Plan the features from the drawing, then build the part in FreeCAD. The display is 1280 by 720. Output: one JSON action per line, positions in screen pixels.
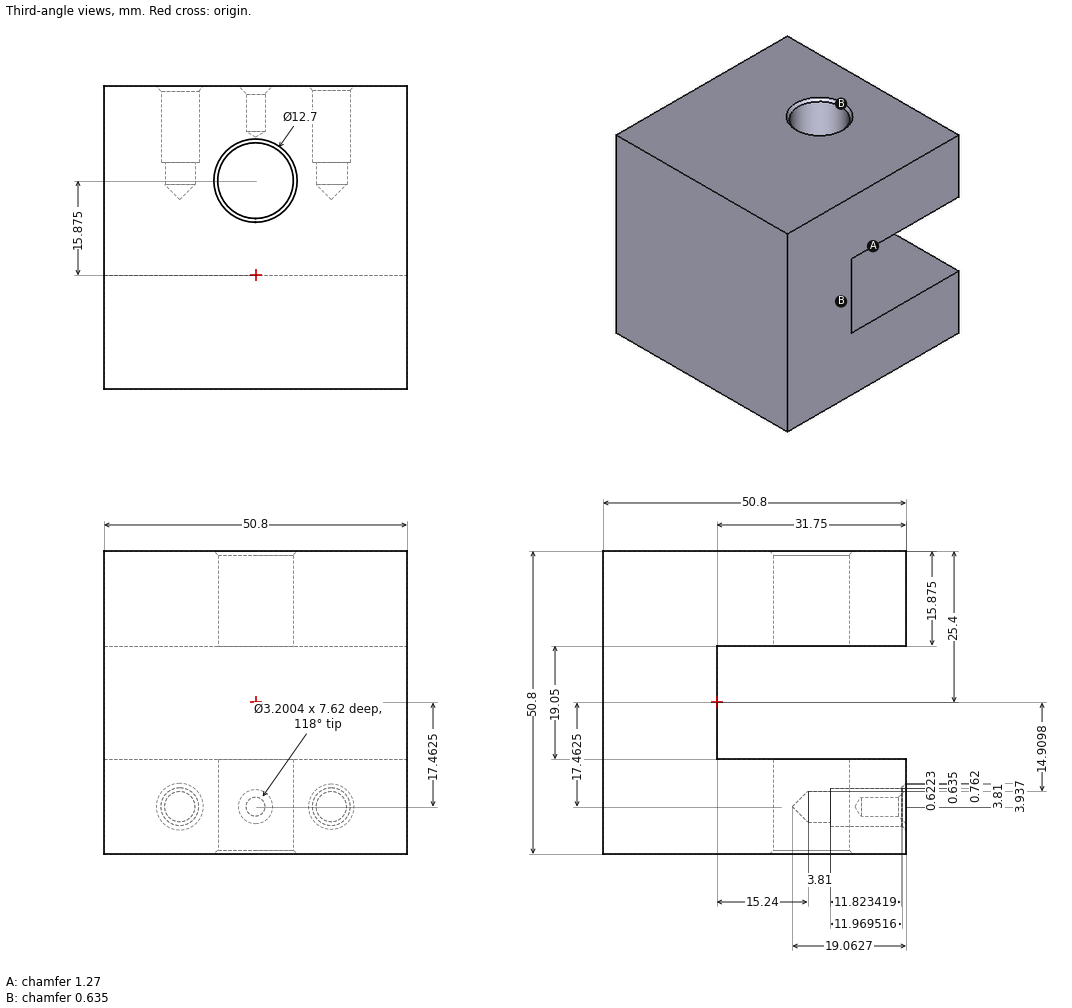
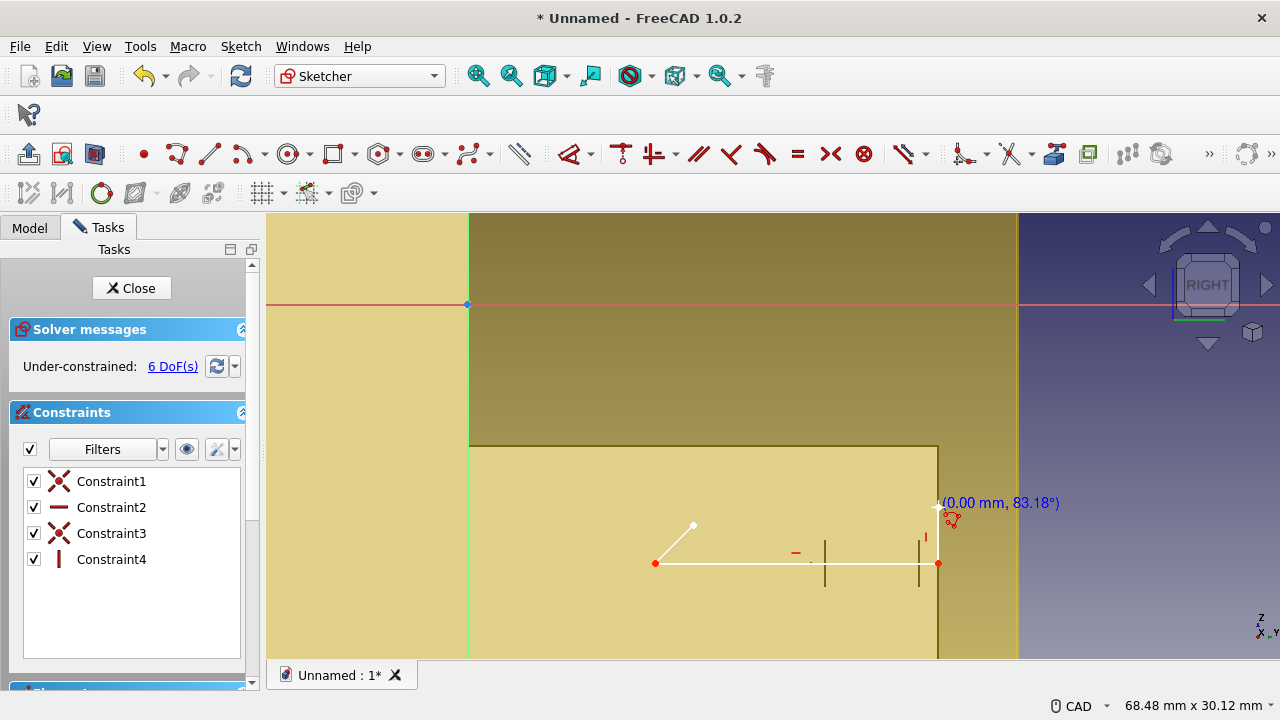
{"action": "scroll", "coordinate": [927, 516], "scroll_direction": "up", "scroll_amount": 2}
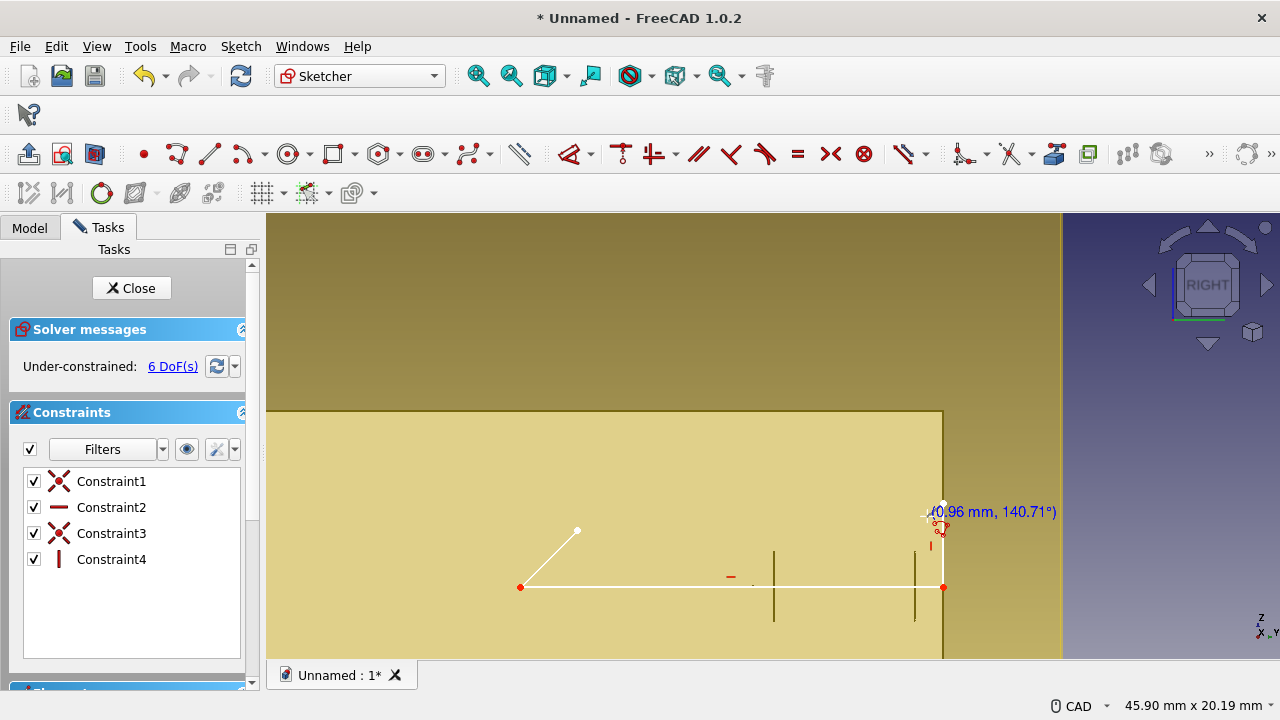
{"action": "left_click", "coordinate": [927, 516]}
{"action": "left_click", "coordinate": [662, 516]}
{"action": "left_click", "coordinate": [662, 530]}
{"action": "left_click", "coordinate": [578, 531]}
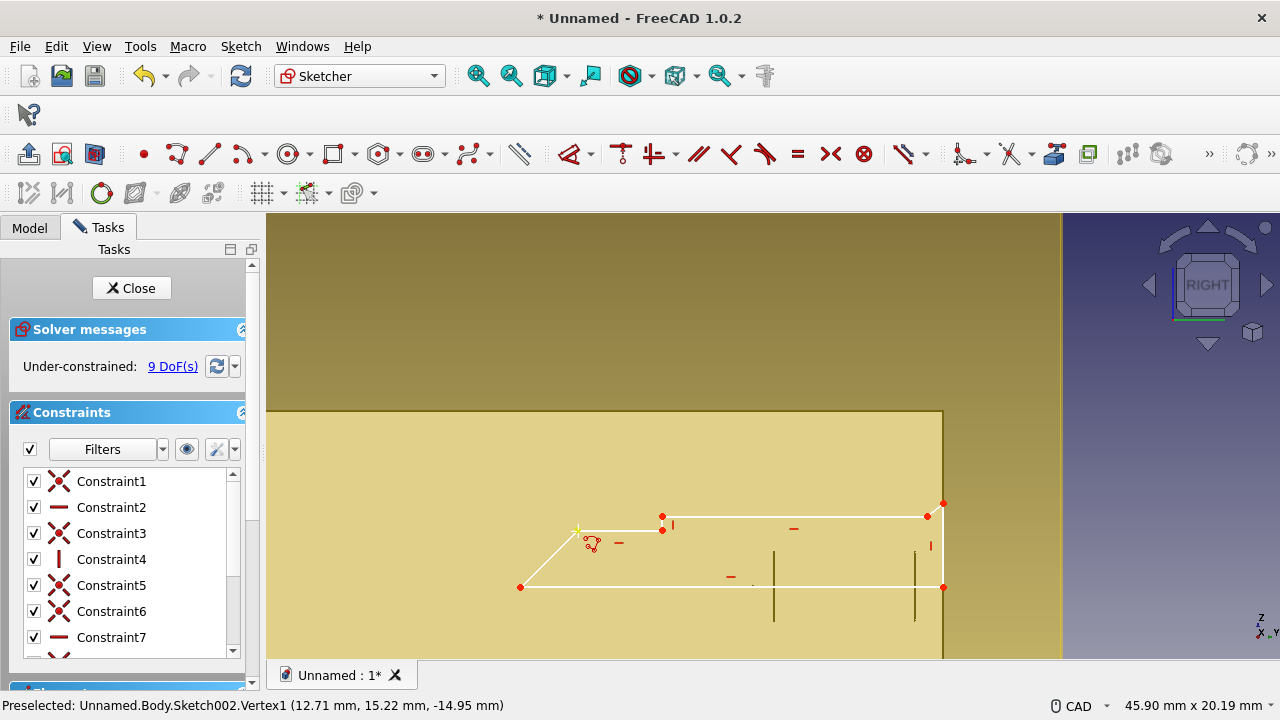
{"action": "left_click", "coordinate": [210, 154]}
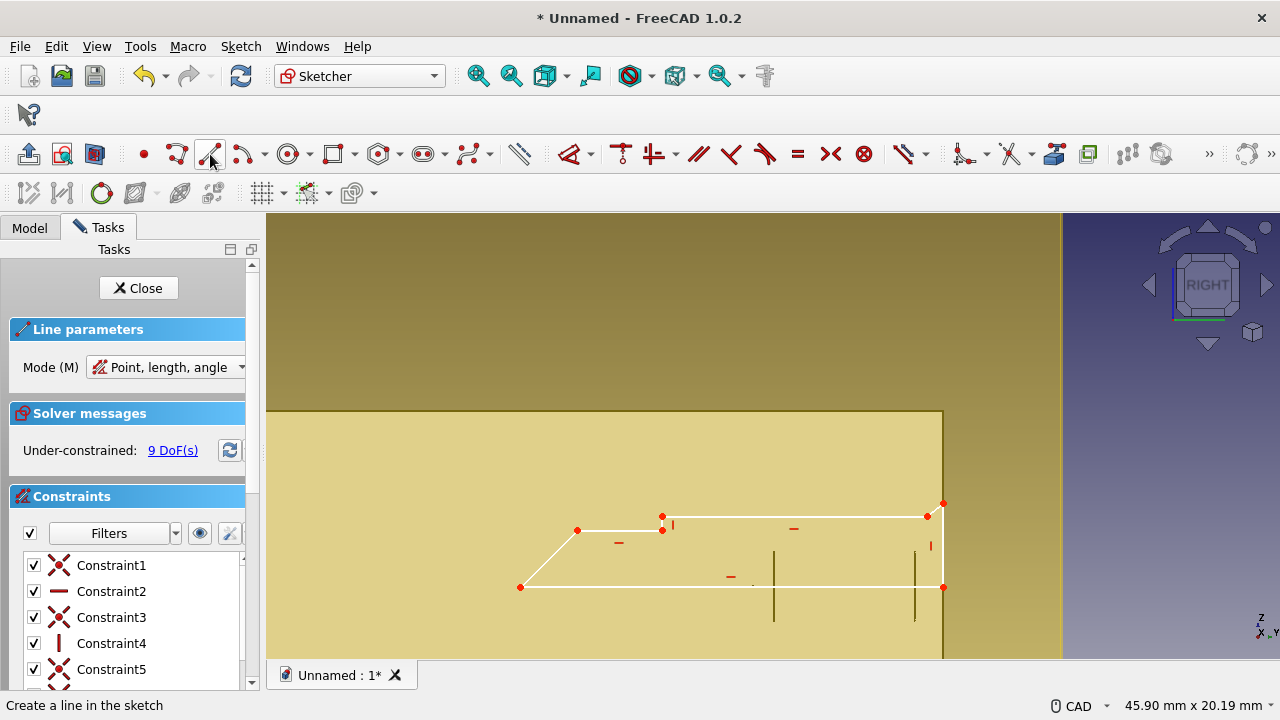
{"action": "left_click", "coordinate": [479, 586]}
{"action": "left_click", "coordinate": [353, 586]}
{"action": "key", "text": "Escape"}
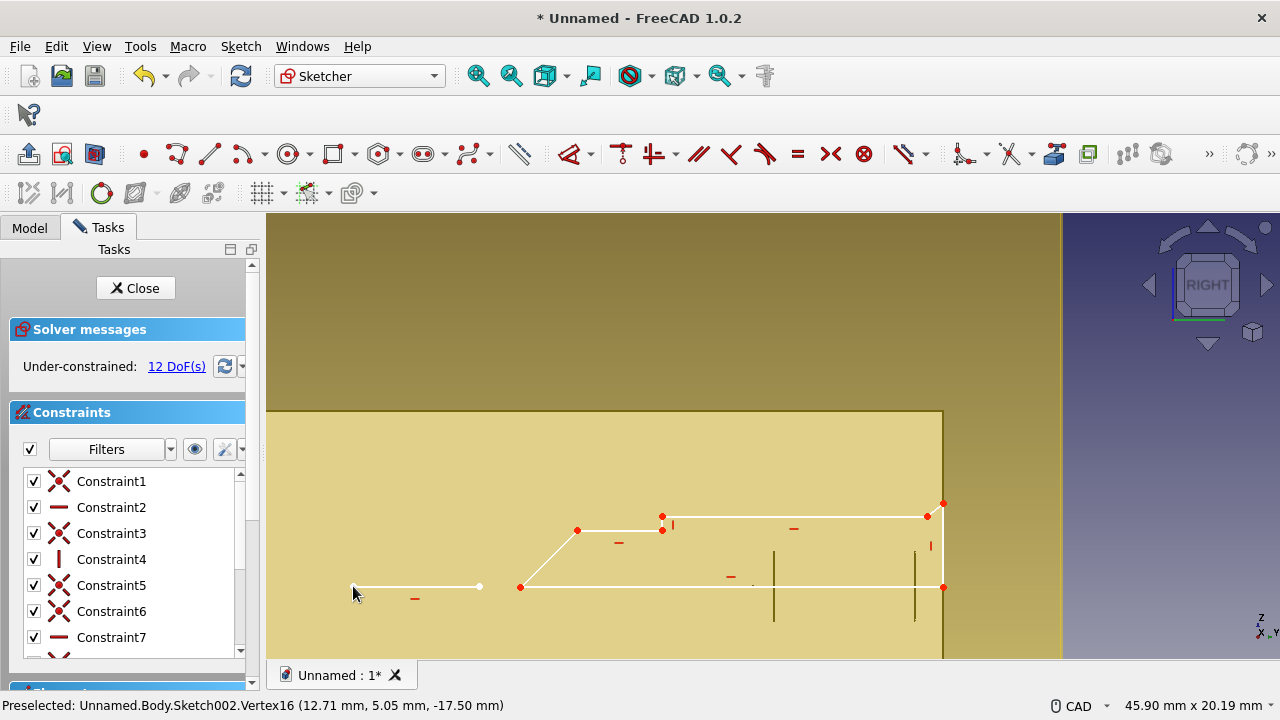
{"action": "left_click", "coordinate": [441, 587]}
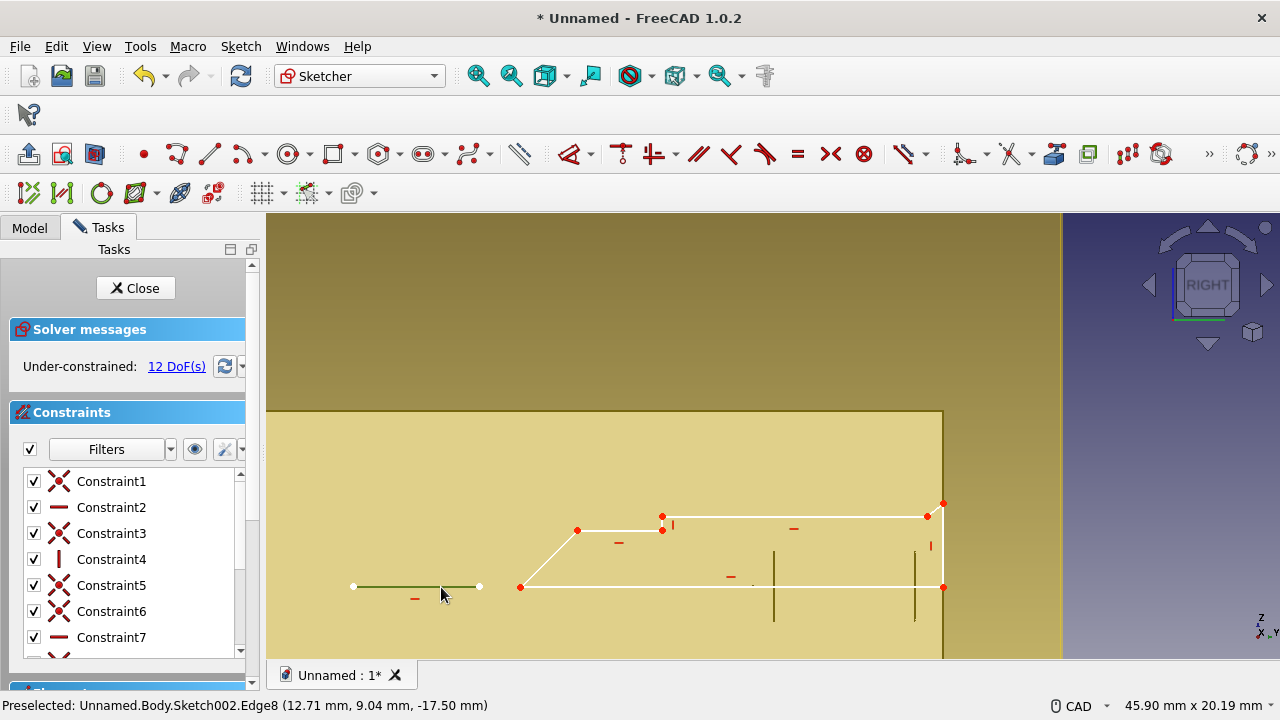
{"action": "left_click", "coordinate": [520, 154]}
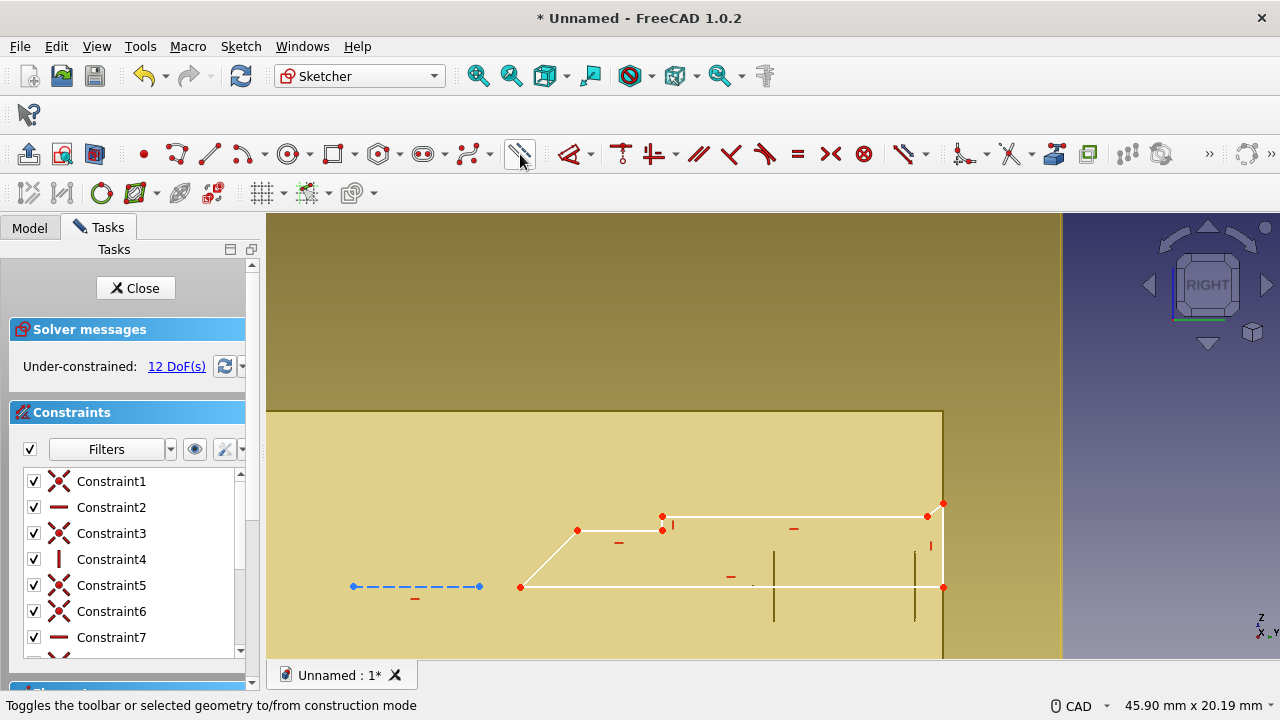
{"action": "left_click", "coordinate": [568, 154]}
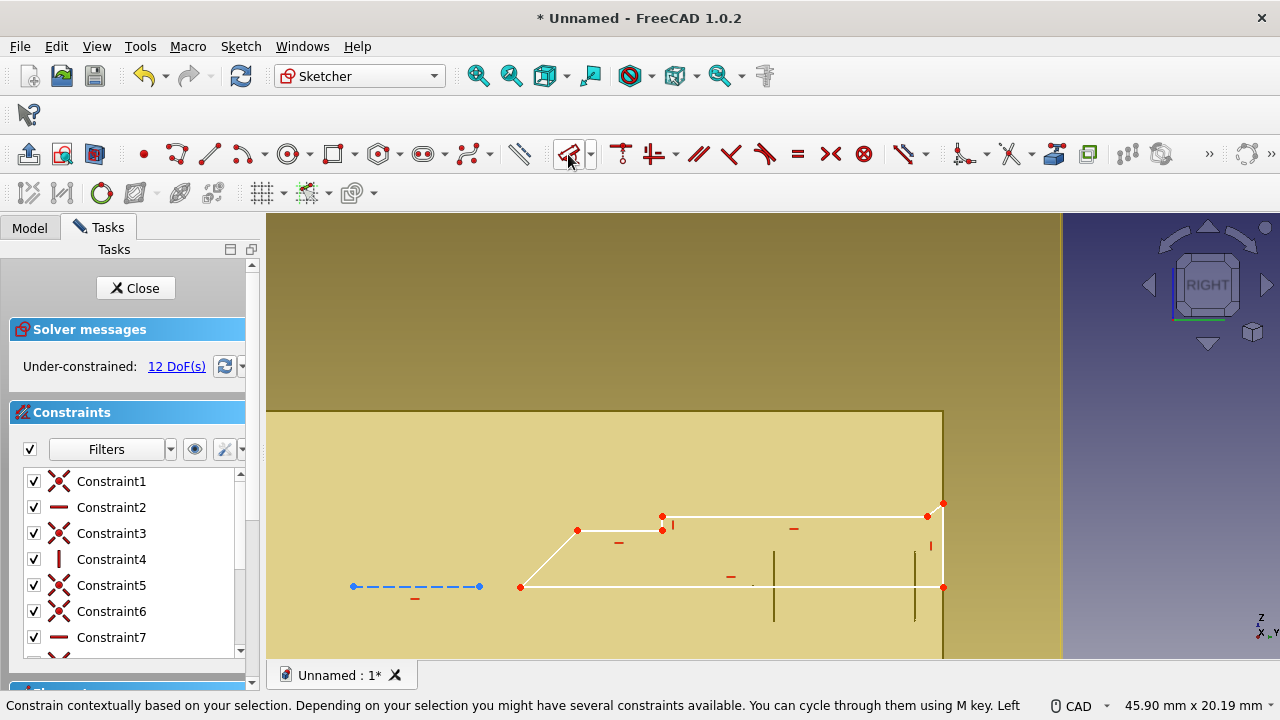
{"action": "left_click", "coordinate": [943, 562]}
{"action": "left_click", "coordinate": [977, 546]}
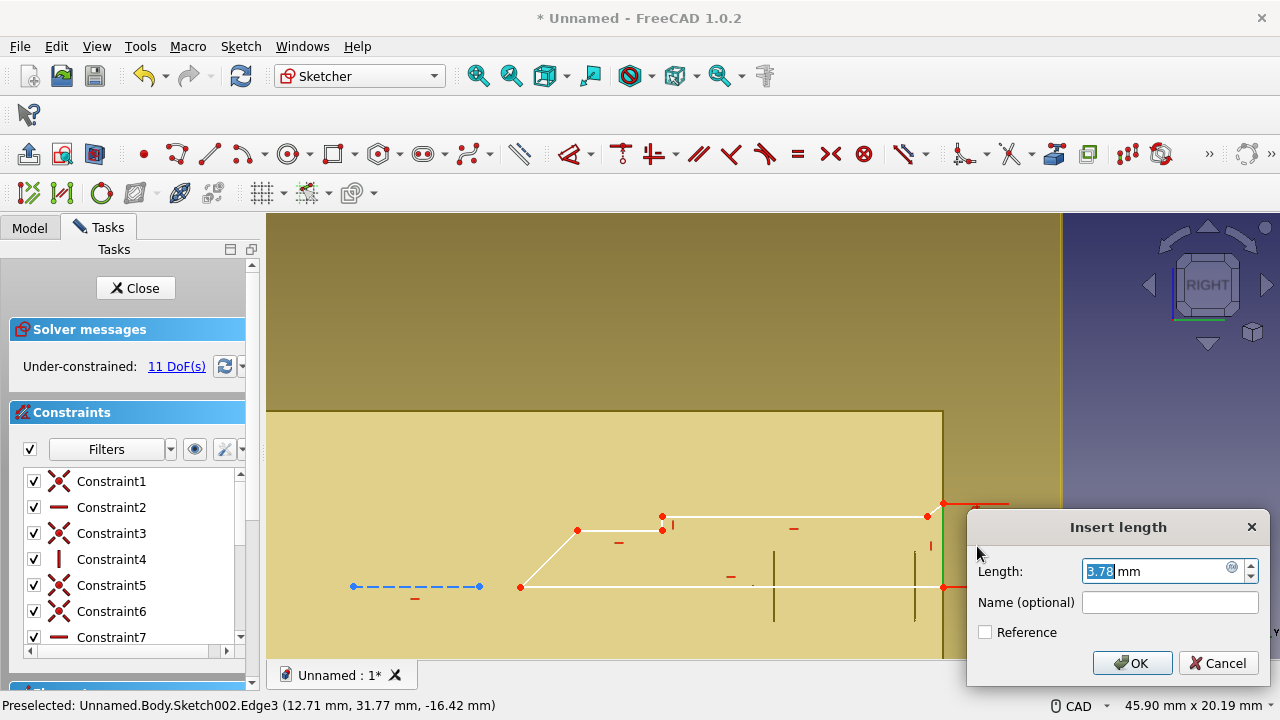
{"action": "type", "text": "3.81"}
{"action": "key", "text": "Return"}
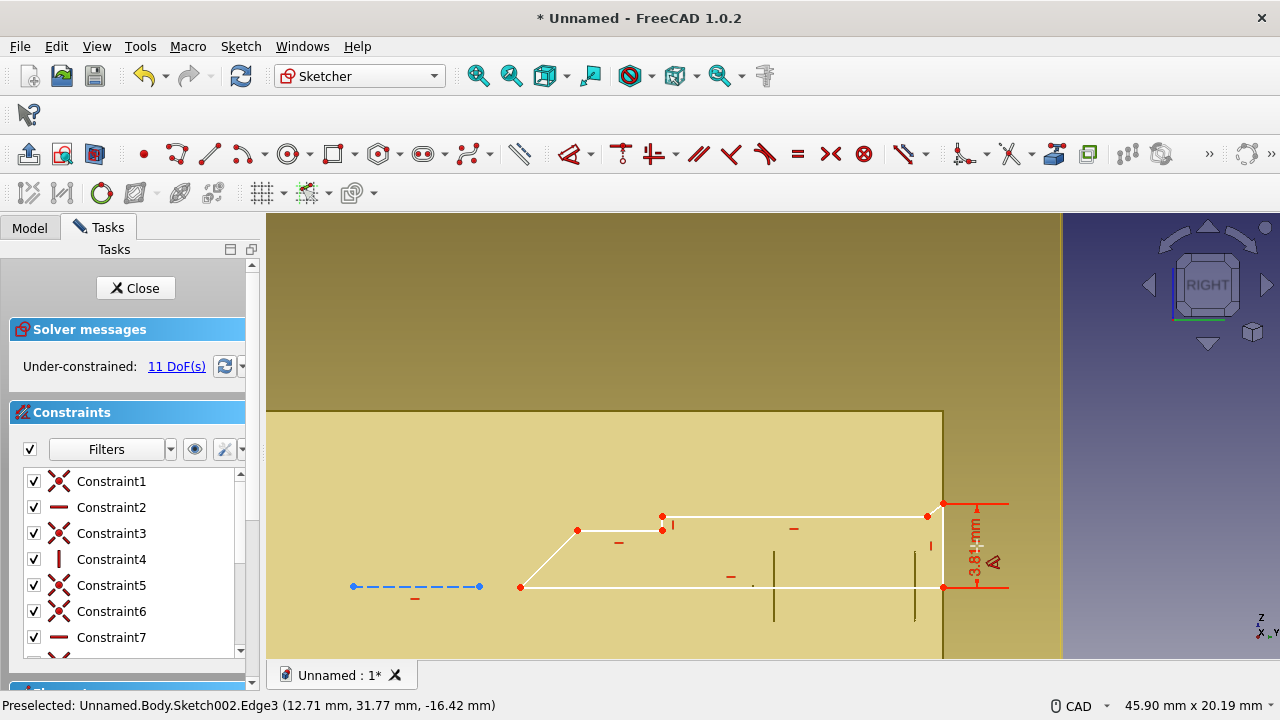
{"action": "left_click", "coordinate": [637, 531]}
{"action": "left_click", "coordinate": [620, 565]}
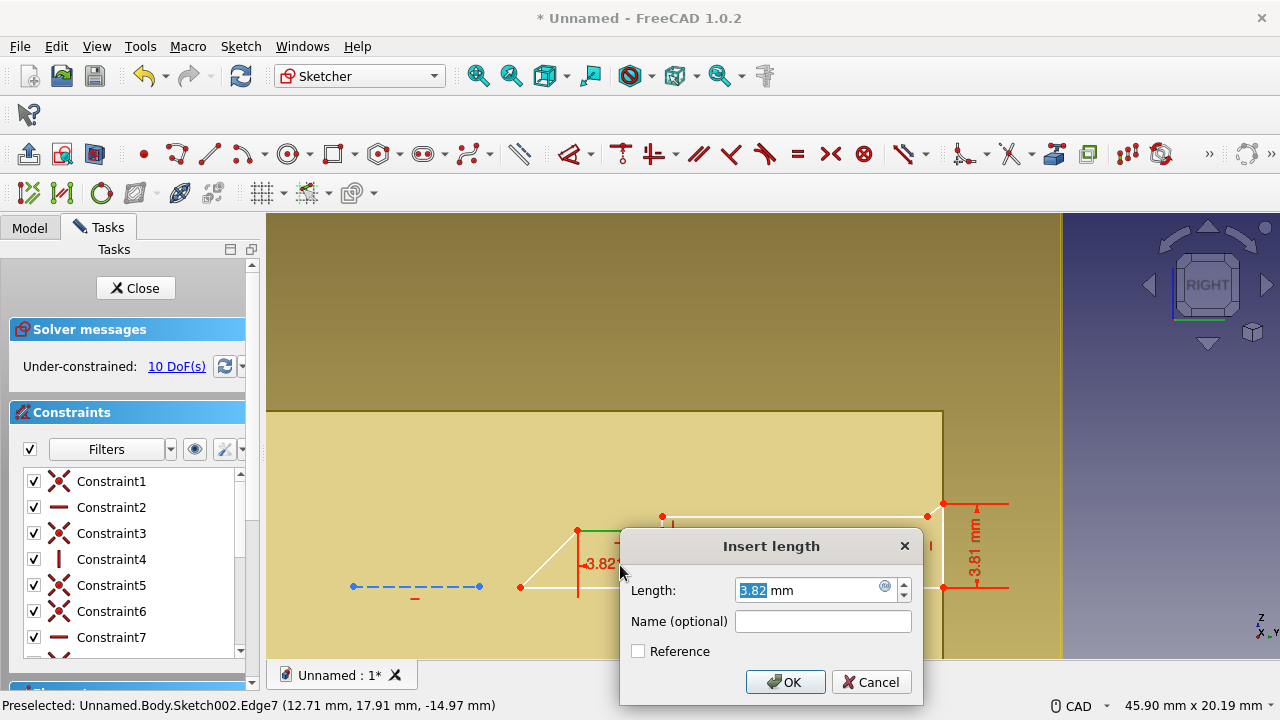
{"action": "type", "text": "3.81"}
{"action": "key", "text": "Return"}